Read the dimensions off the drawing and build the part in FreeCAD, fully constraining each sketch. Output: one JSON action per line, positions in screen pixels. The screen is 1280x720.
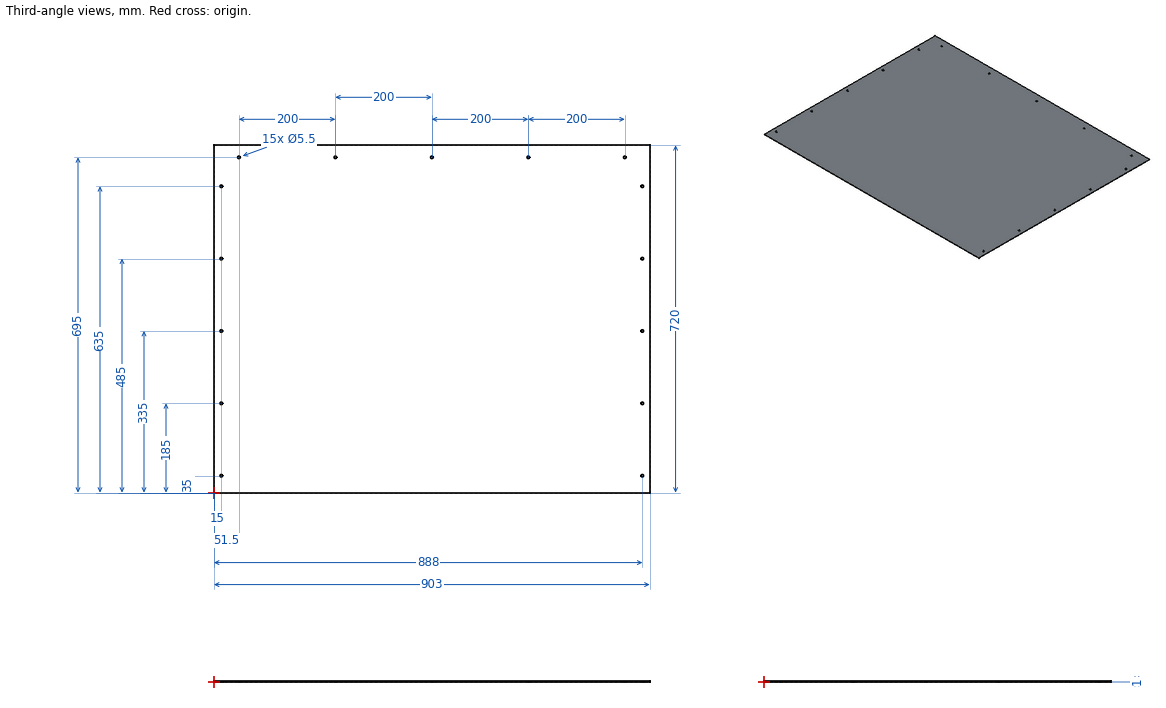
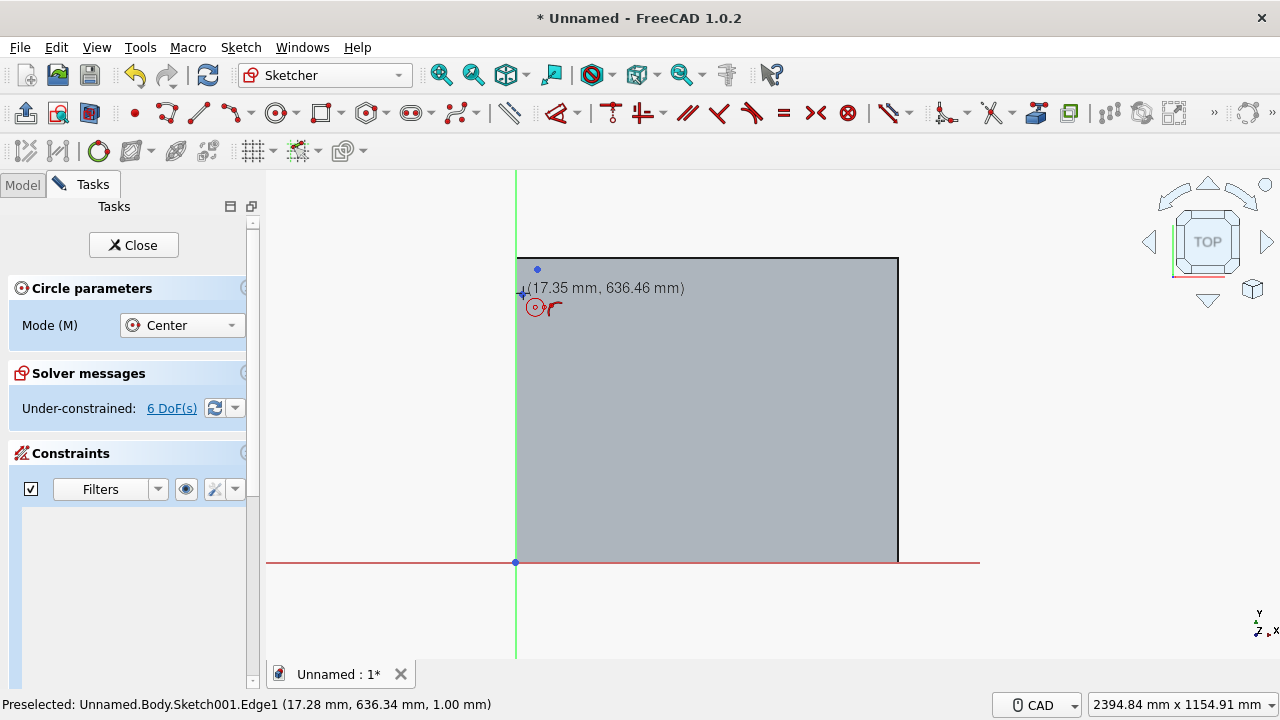
{"action": "scroll", "coordinate": [622, 269], "scroll_direction": "up", "scroll_amount": 15}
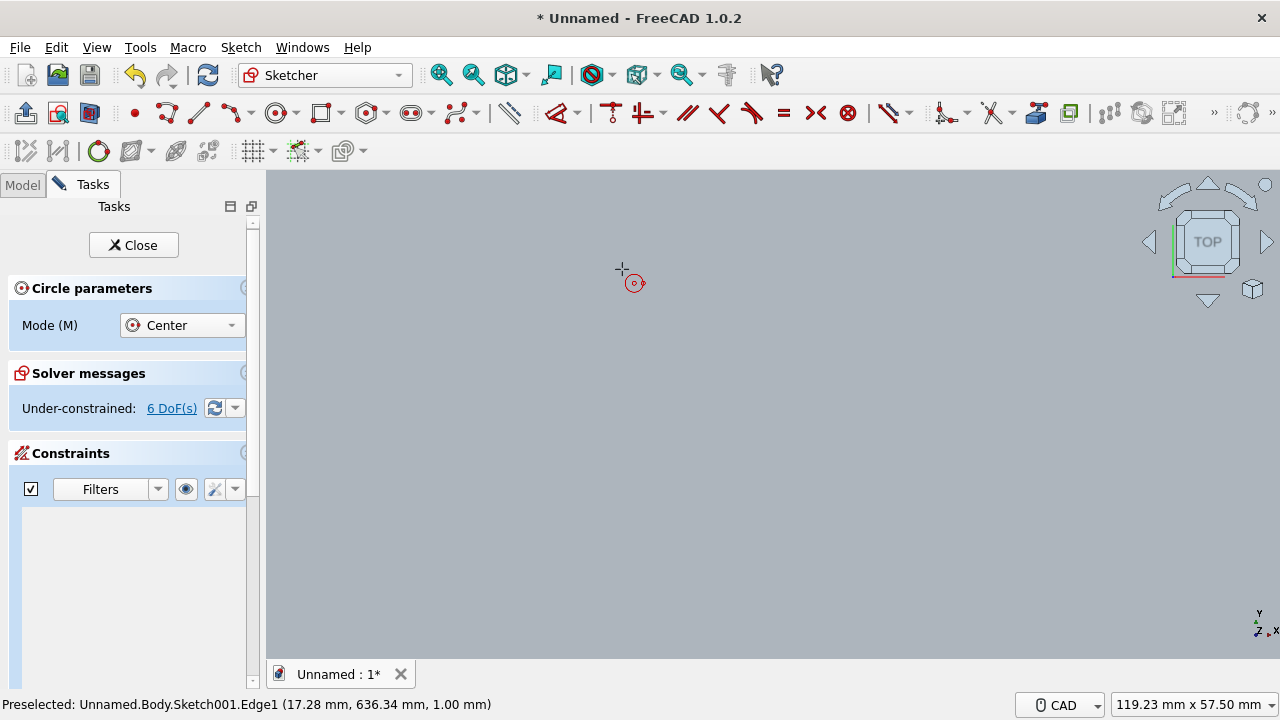
{"action": "scroll", "coordinate": [622, 269], "scroll_direction": "down", "scroll_amount": 15}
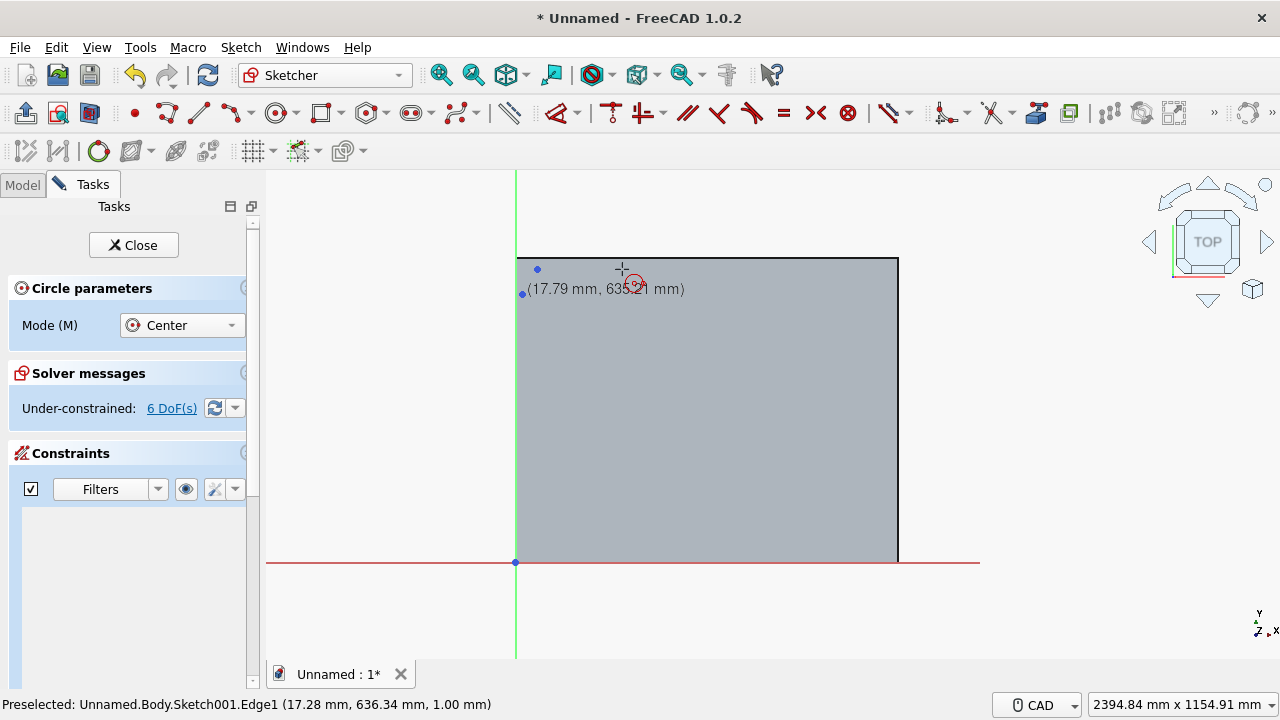
{"action": "left_click", "coordinate": [622, 269]}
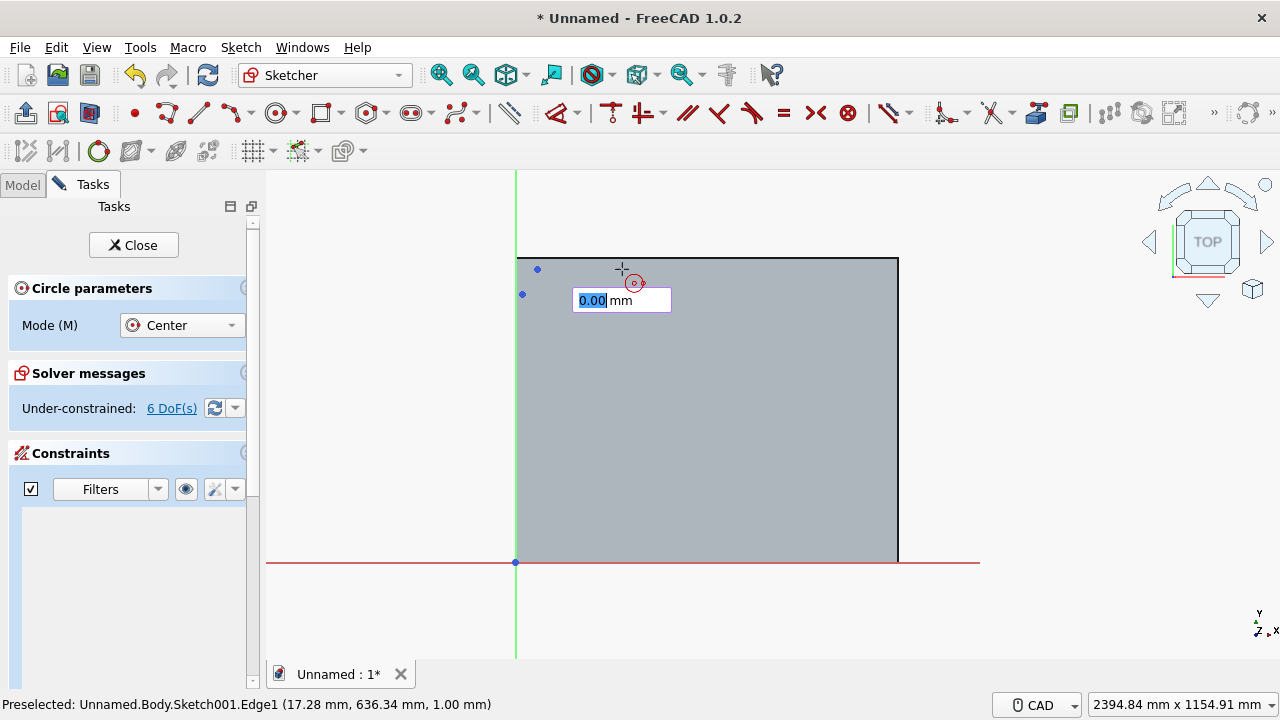
{"action": "scroll", "coordinate": [623, 268], "scroll_direction": "up", "scroll_amount": 14}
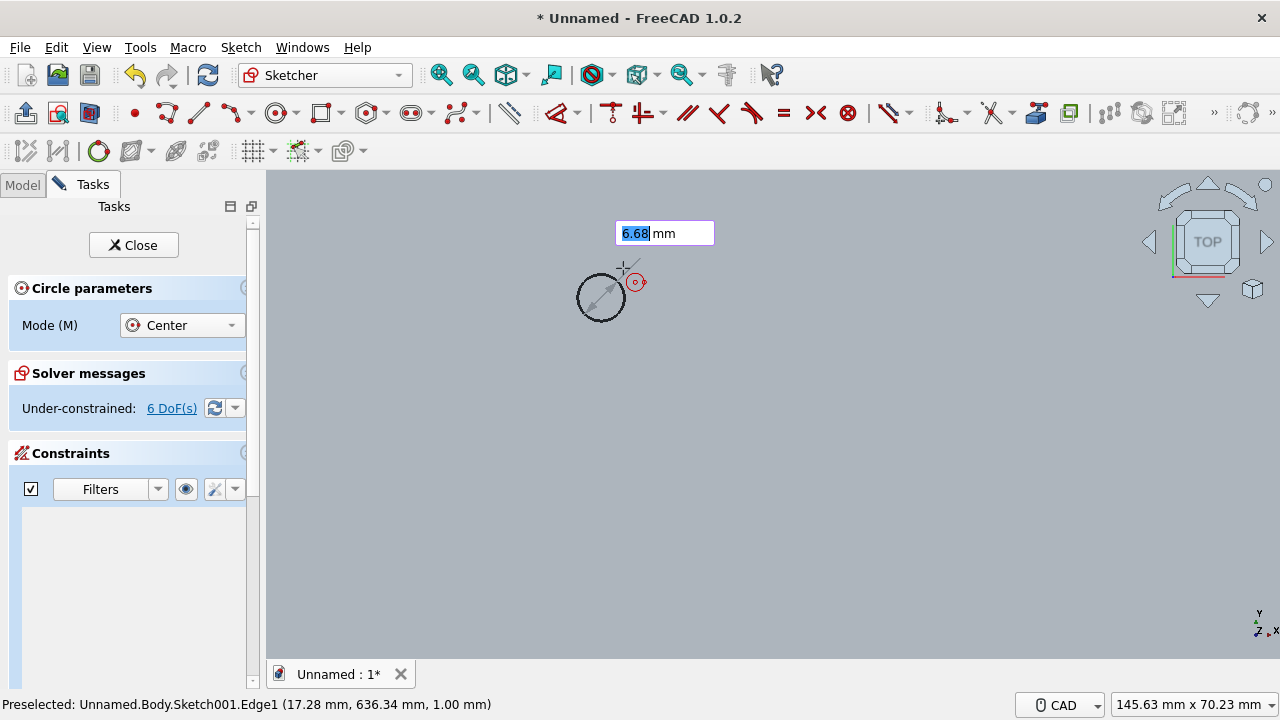
{"action": "left_click", "coordinate": [621, 260]}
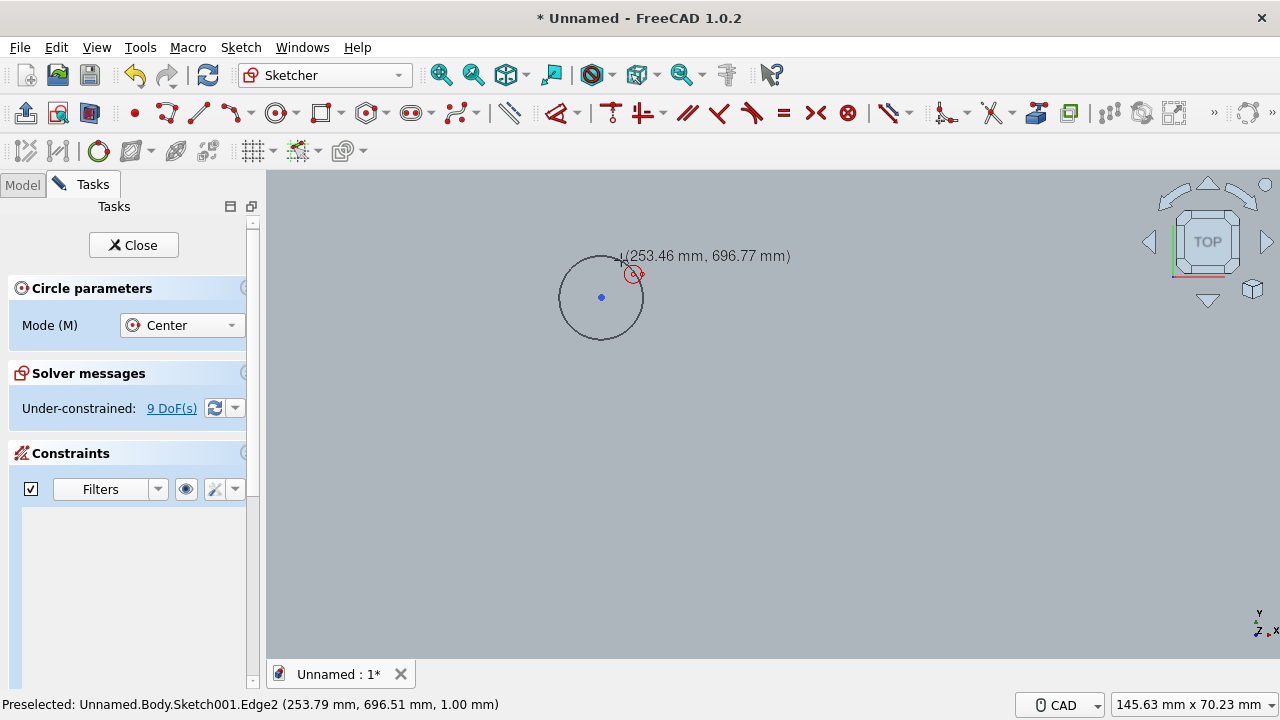
{"action": "scroll", "coordinate": [623, 268], "scroll_direction": "down", "scroll_amount": 14}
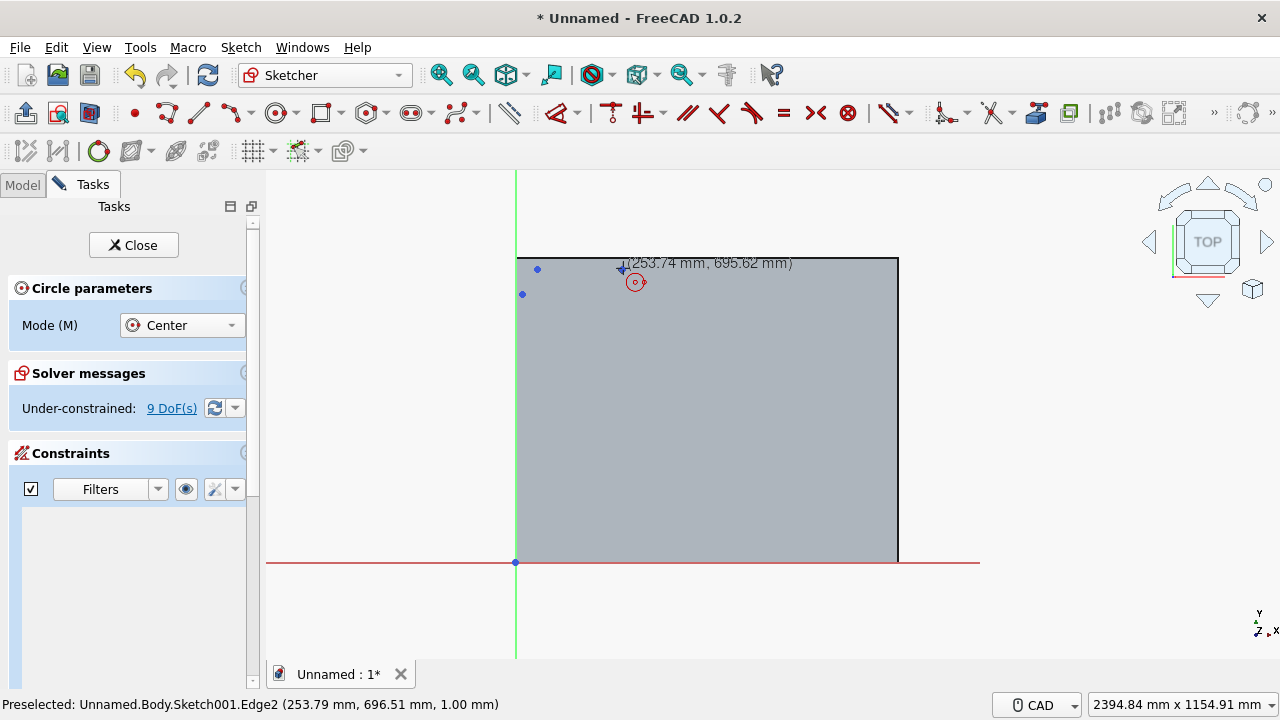
{"action": "scroll", "coordinate": [707, 269], "scroll_direction": "up", "scroll_amount": 15}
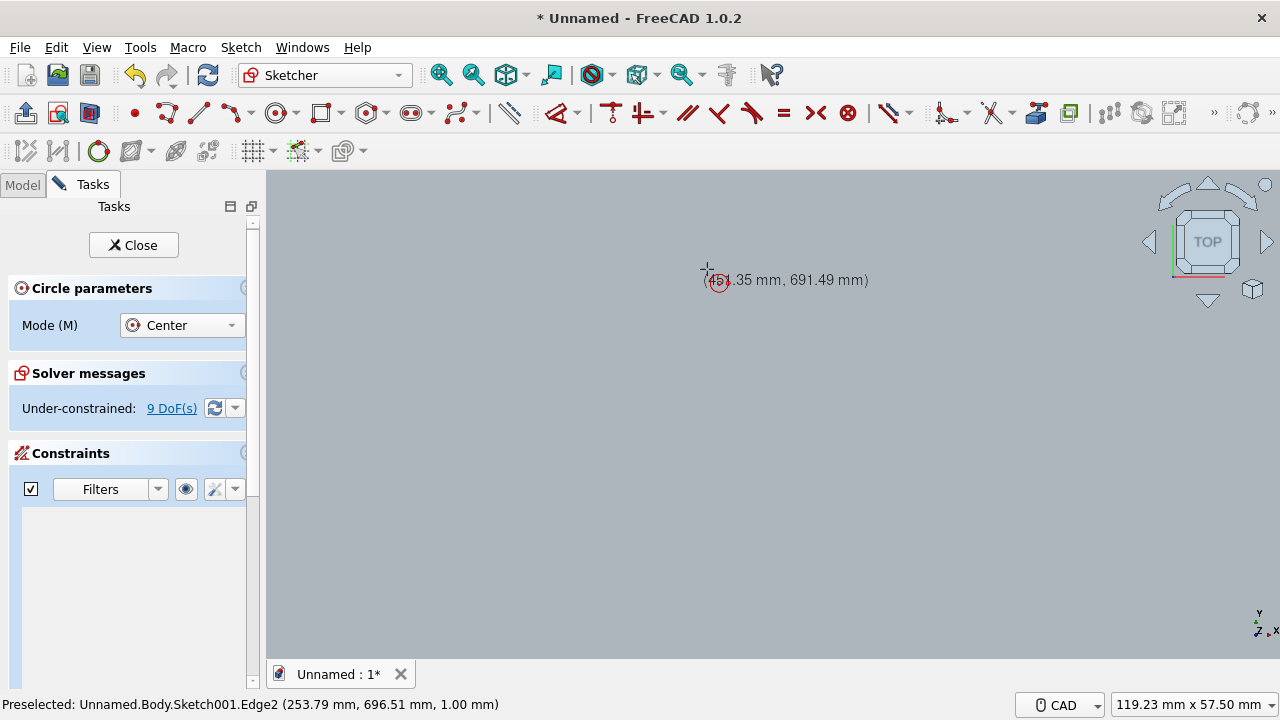
{"action": "scroll", "coordinate": [707, 269], "scroll_direction": "down", "scroll_amount": 15}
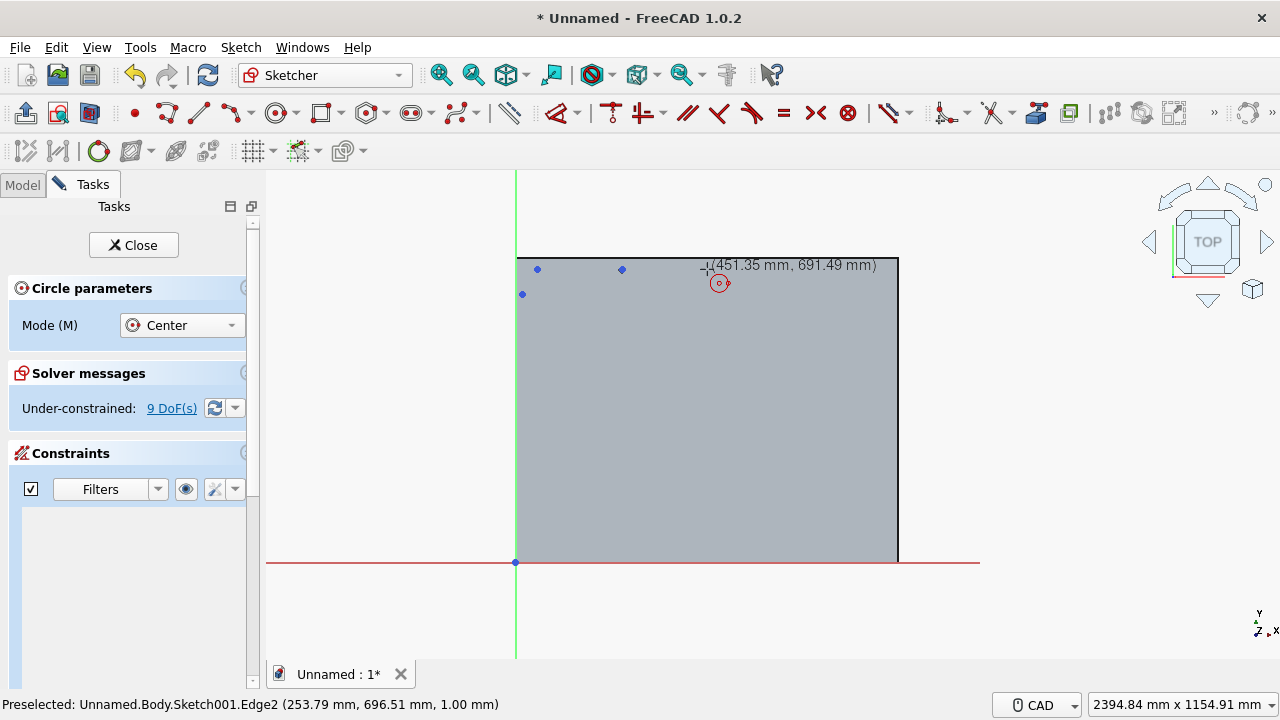
{"action": "left_click", "coordinate": [707, 269]}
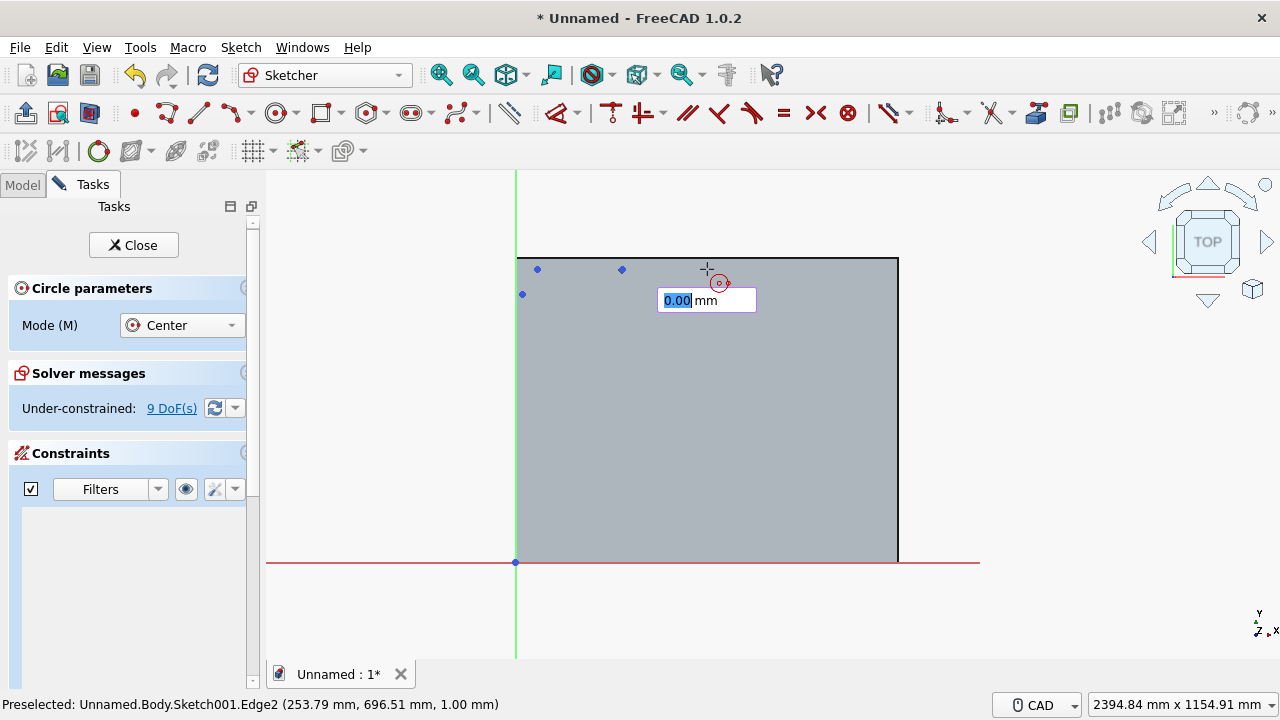
{"action": "scroll", "coordinate": [708, 268], "scroll_direction": "up", "scroll_amount": 14}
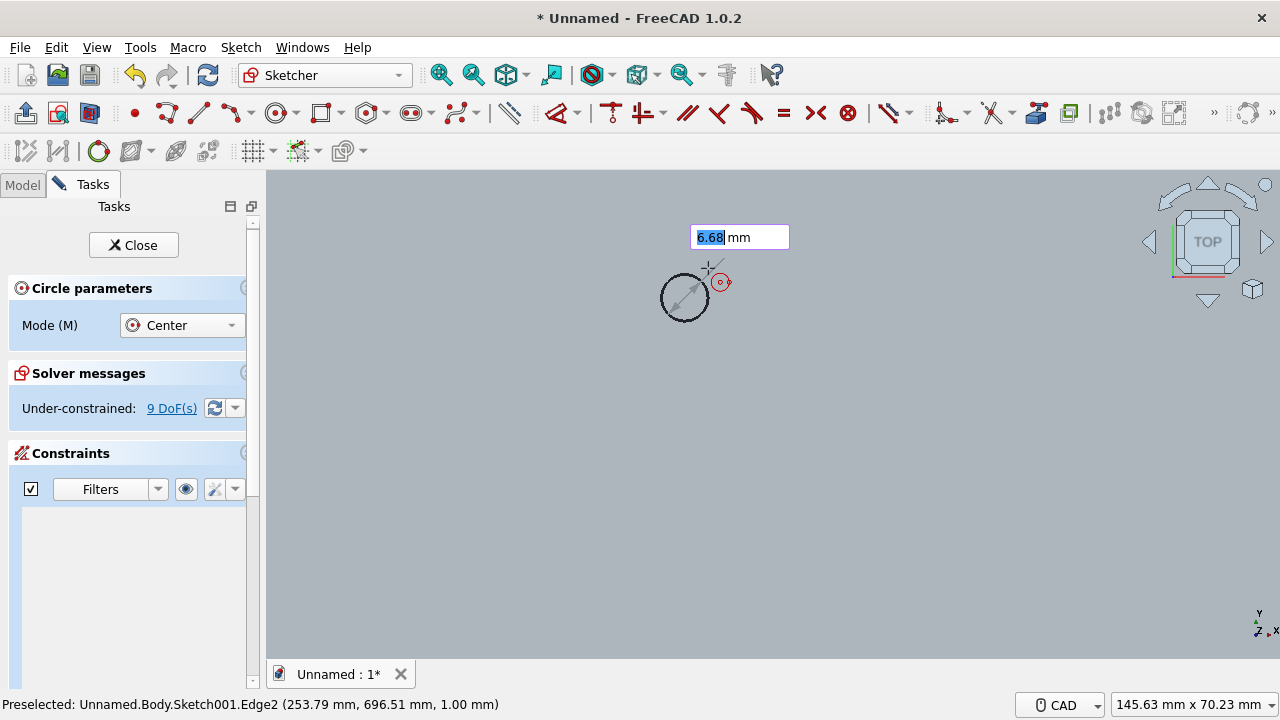
{"action": "left_click", "coordinate": [699, 260]}